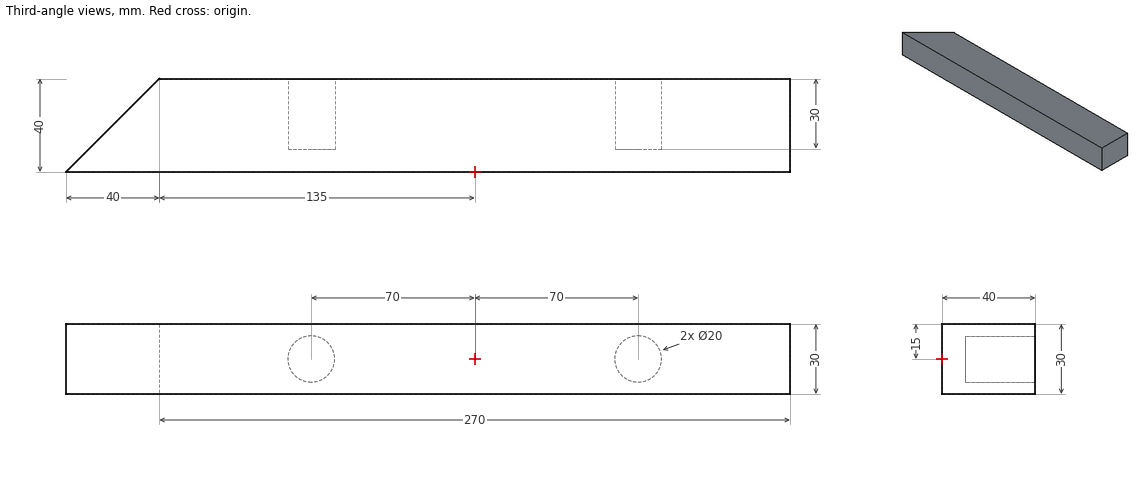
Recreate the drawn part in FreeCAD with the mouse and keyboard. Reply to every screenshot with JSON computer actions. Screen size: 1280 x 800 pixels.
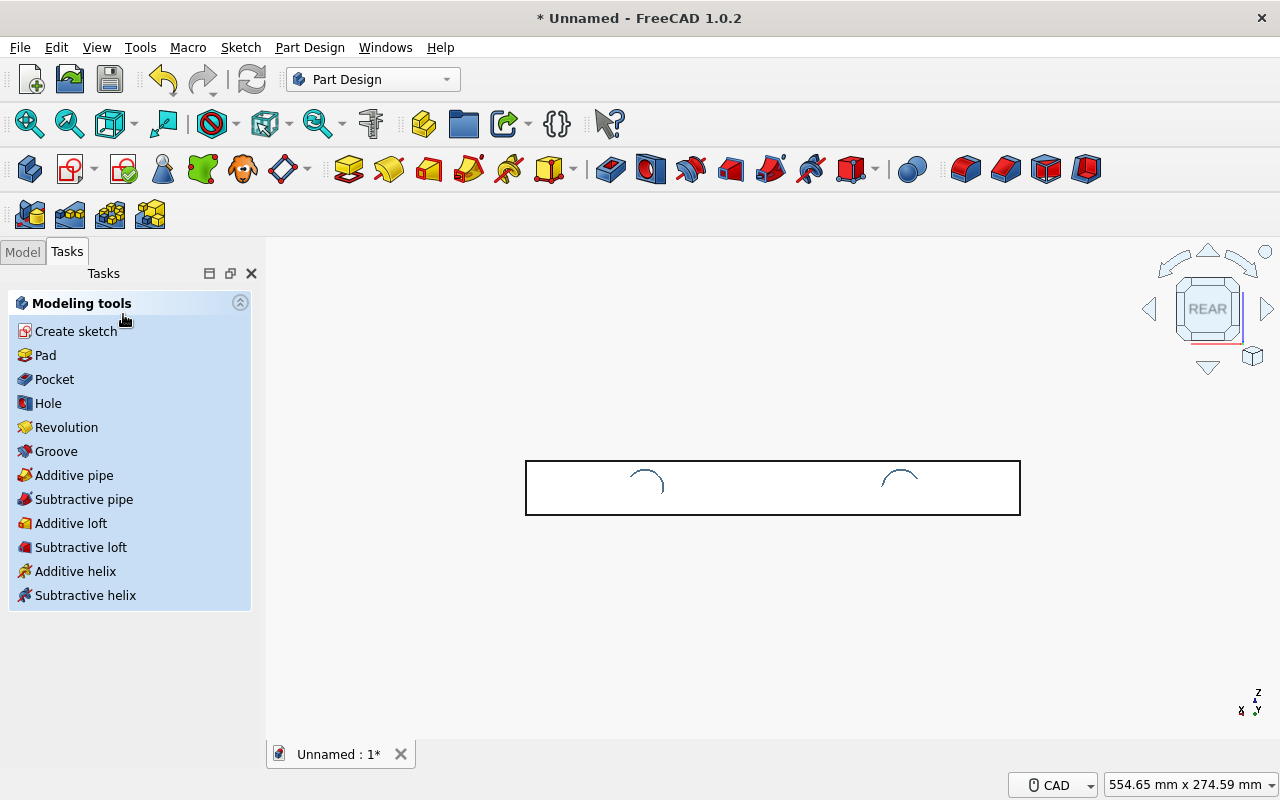
{"action": "left_click", "coordinate": [612, 170]}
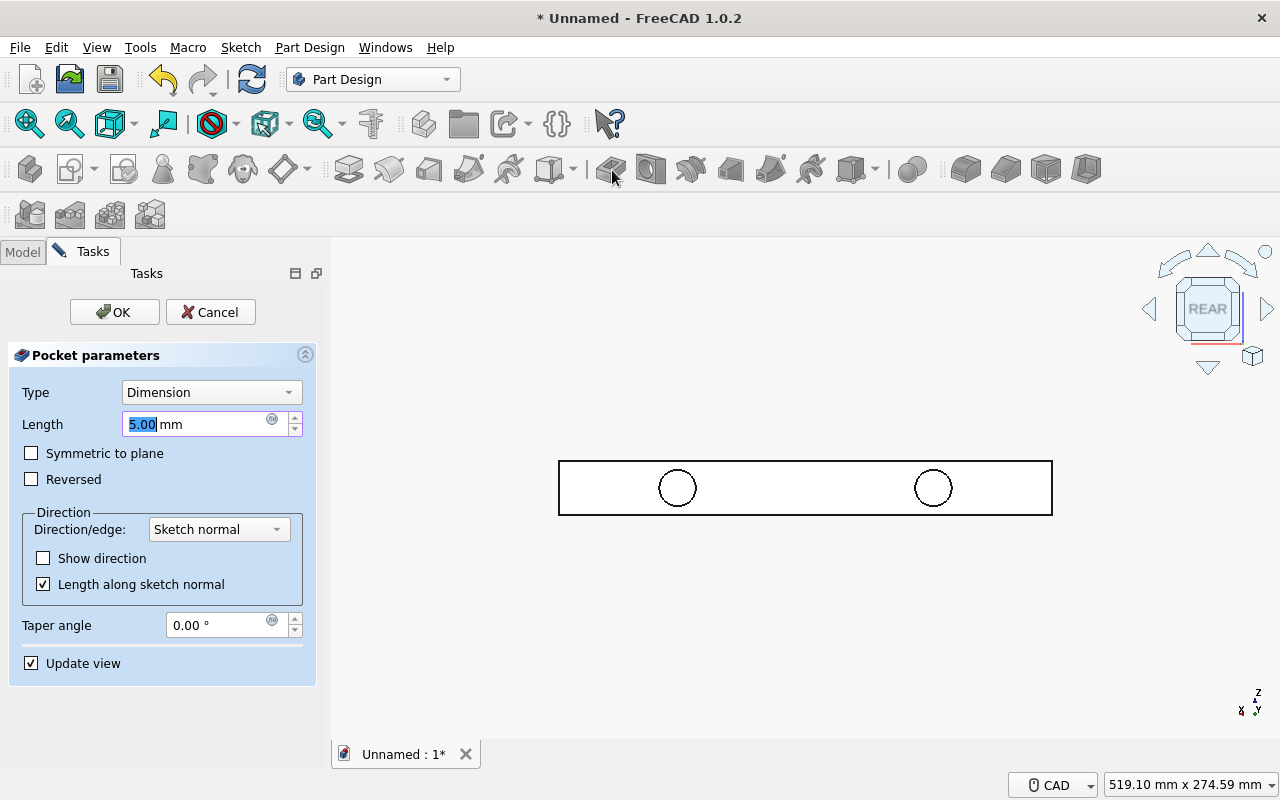
{"action": "type", "text": "30"}
{"action": "key", "text": "Tab"}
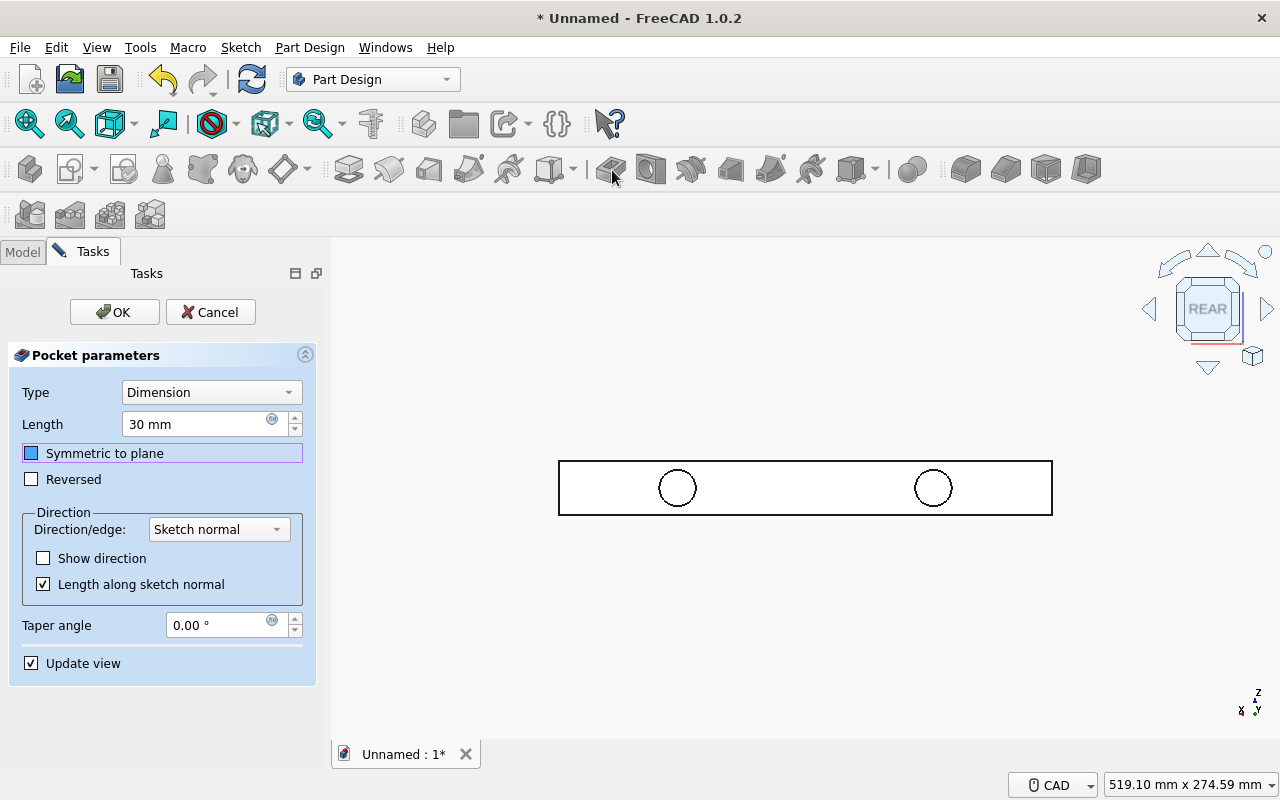
{"action": "left_click", "coordinate": [115, 312]}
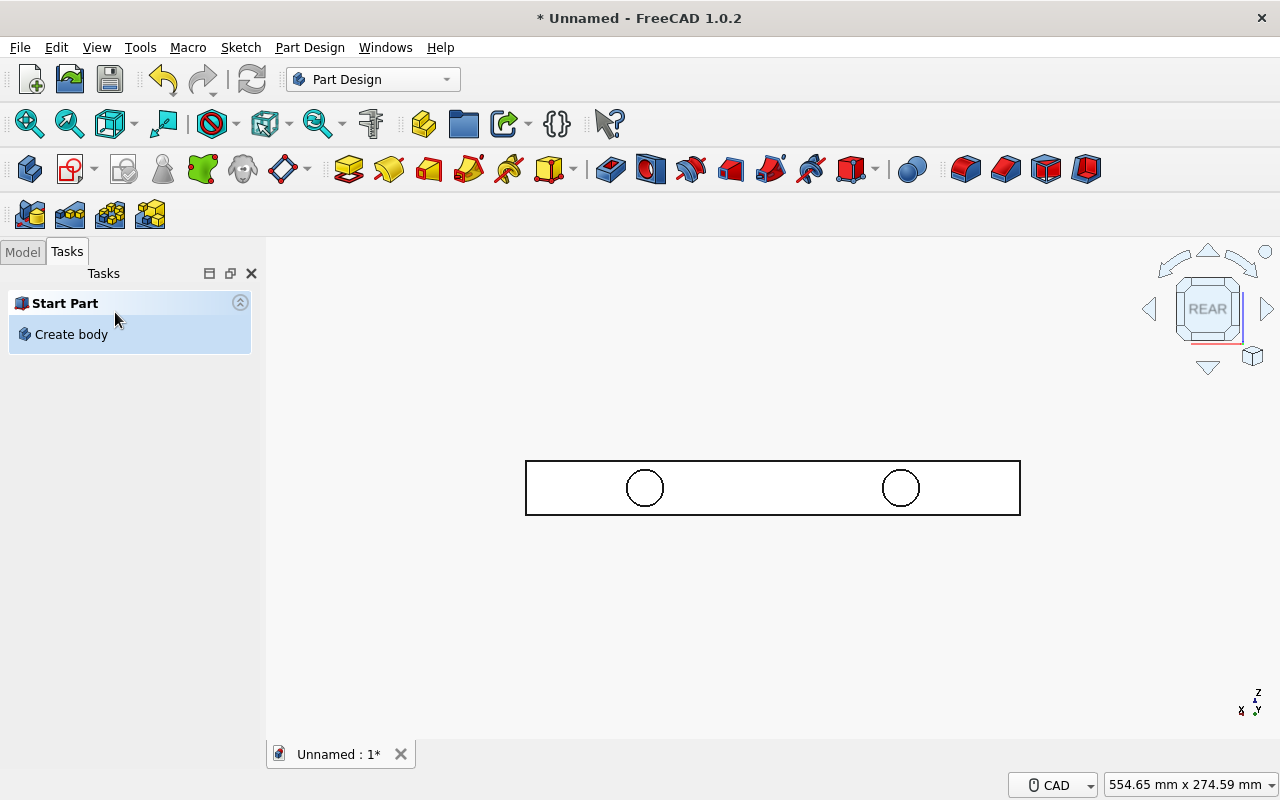
{"action": "key", "text": "6"}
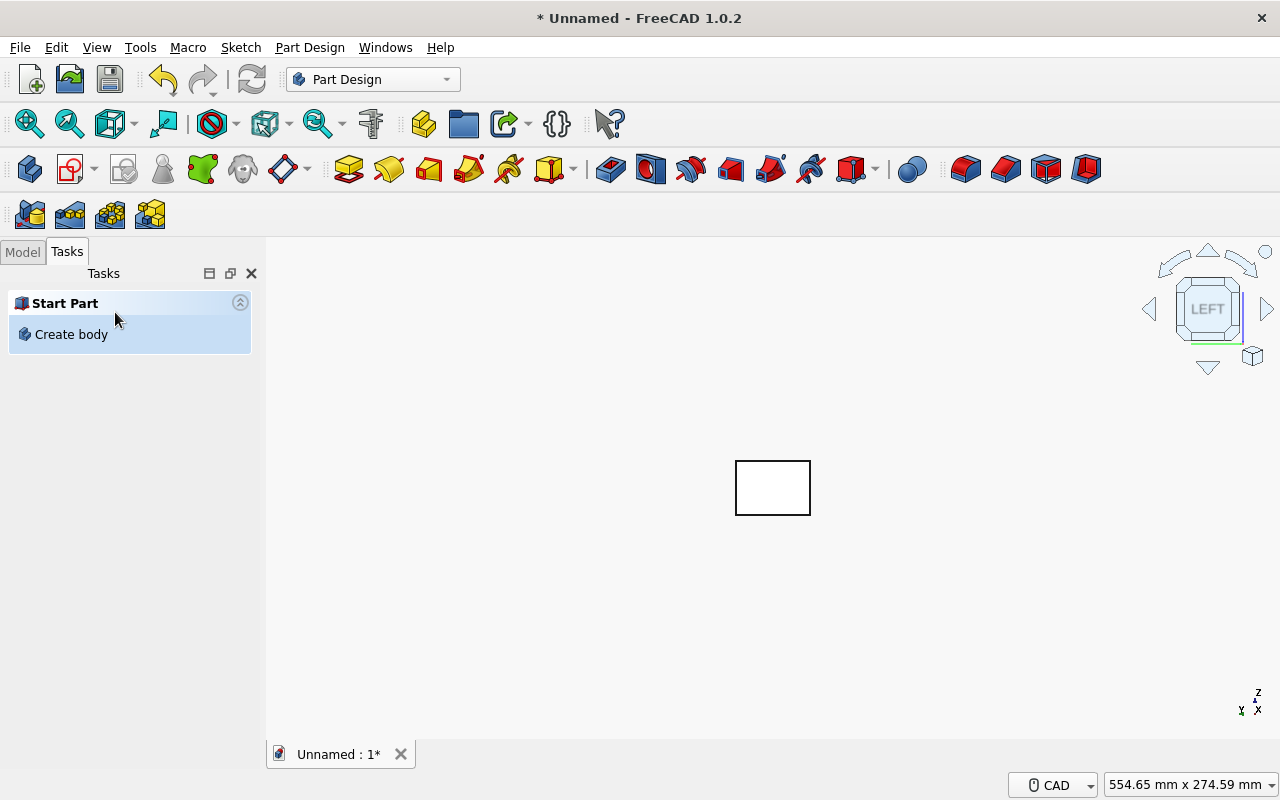
{"action": "left_click", "coordinate": [30, 124]}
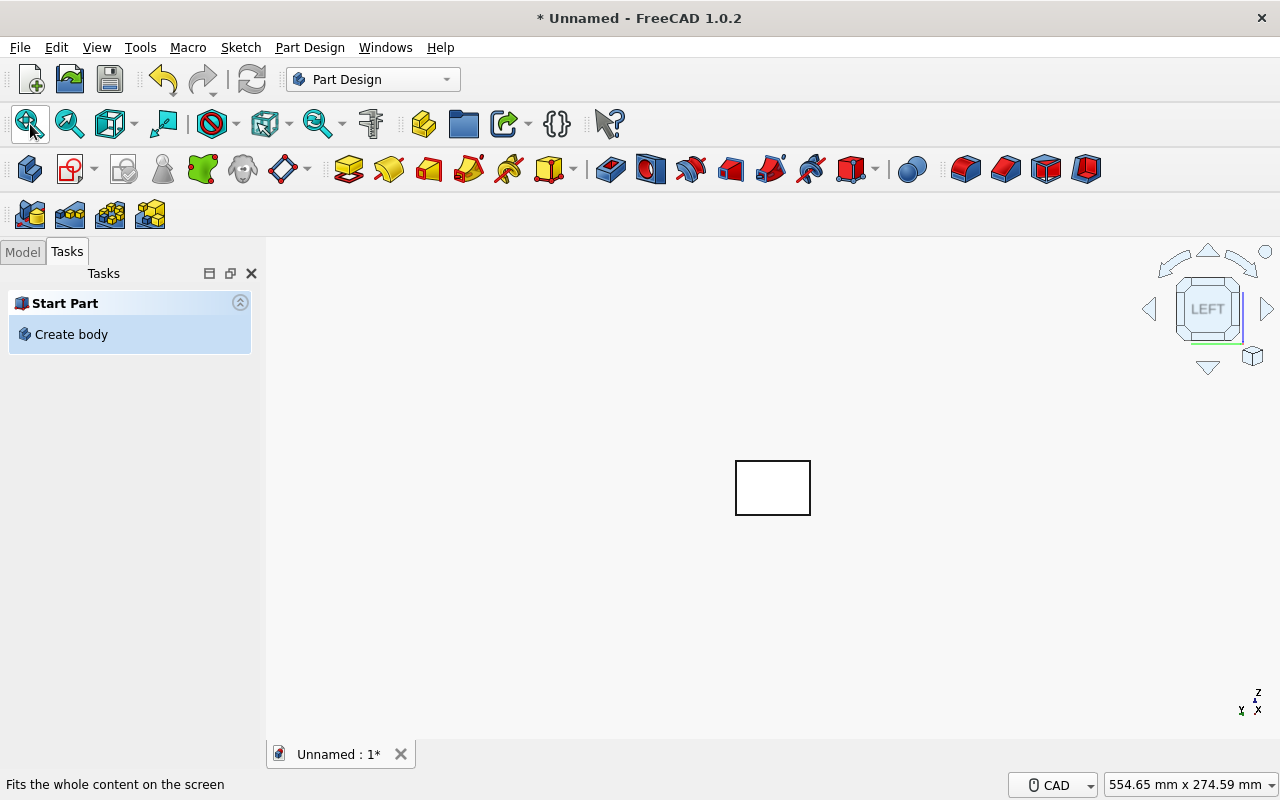
{"action": "left_click", "coordinate": [773, 487]}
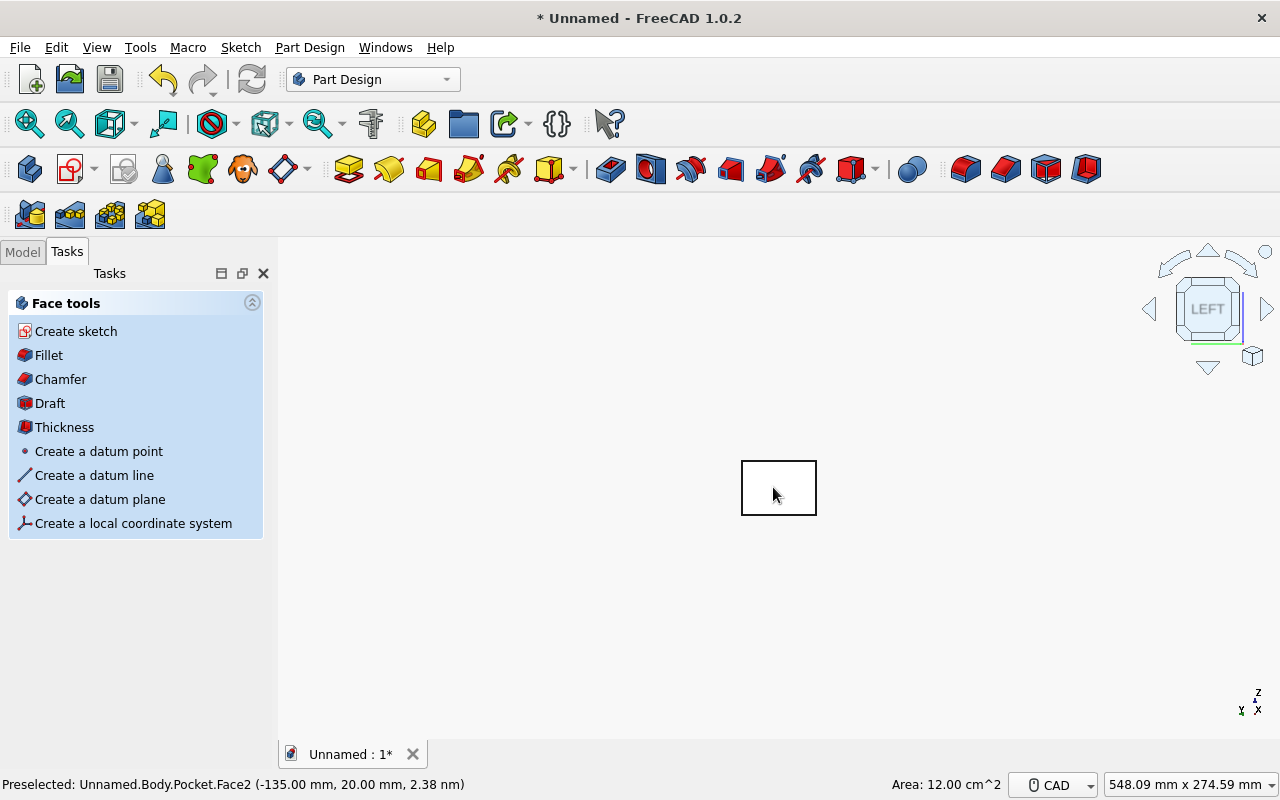
{"action": "left_click", "coordinate": [70, 170]}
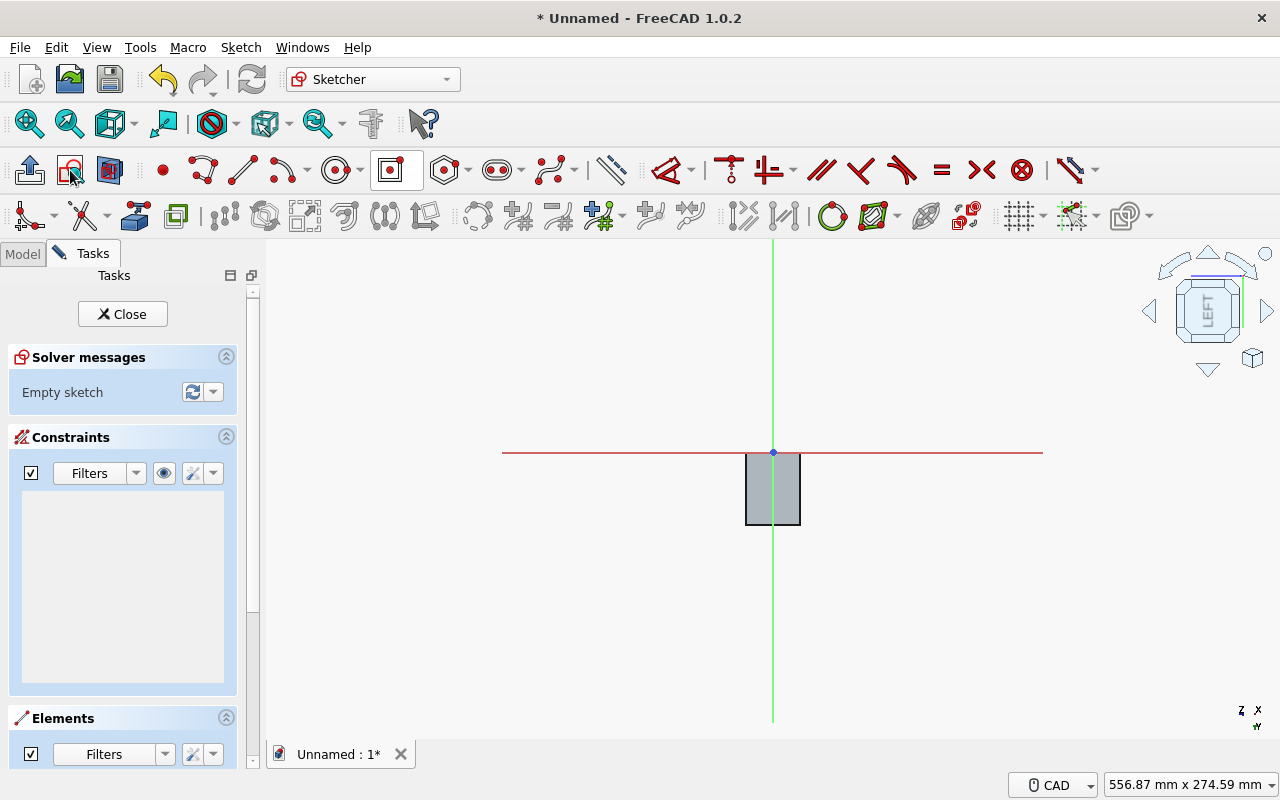
{"action": "scroll", "coordinate": [795, 489], "scroll_direction": "up", "scroll_amount": 7}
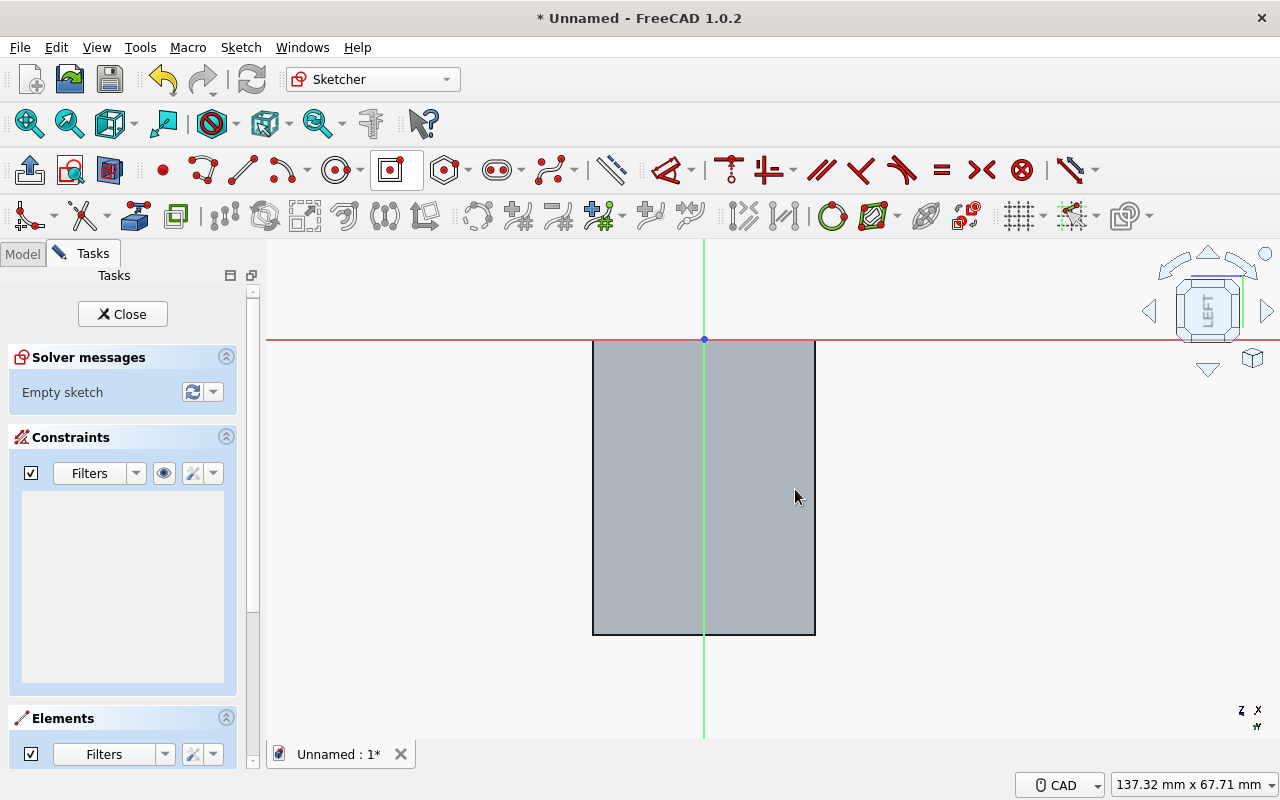
{"action": "left_click", "coordinate": [418, 170]}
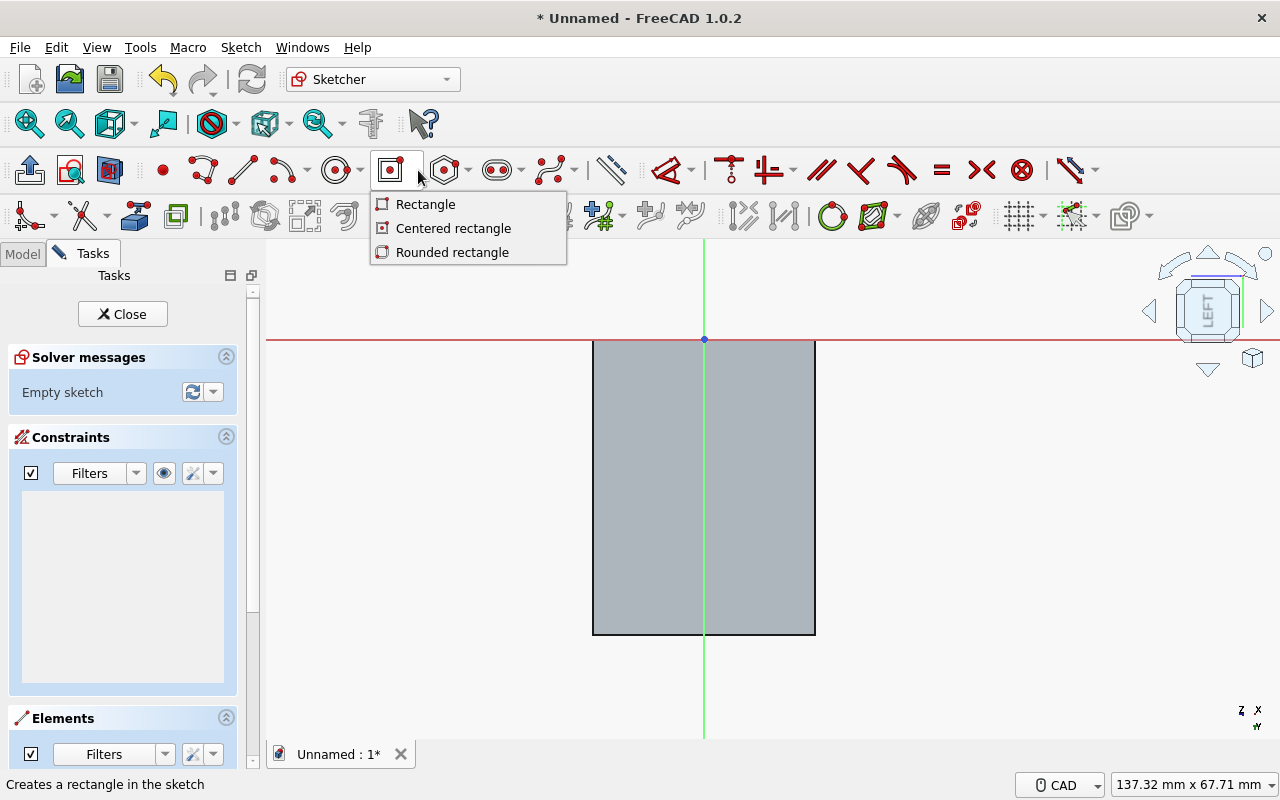
{"action": "left_click", "coordinate": [468, 204]}